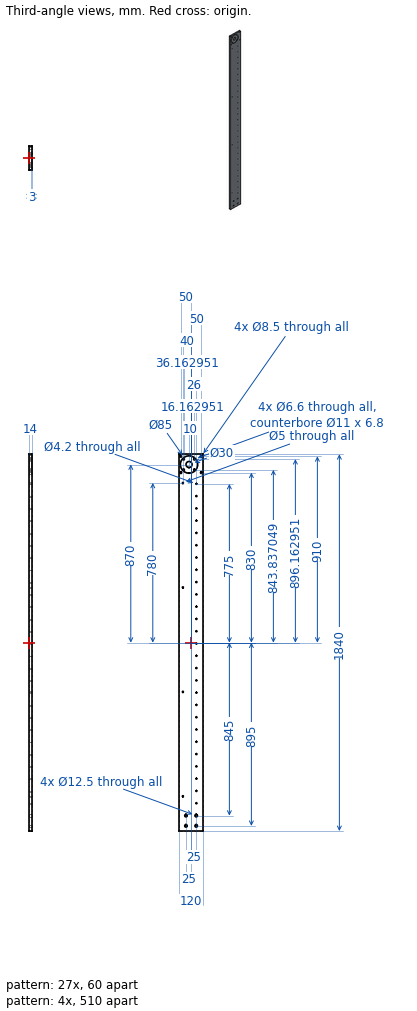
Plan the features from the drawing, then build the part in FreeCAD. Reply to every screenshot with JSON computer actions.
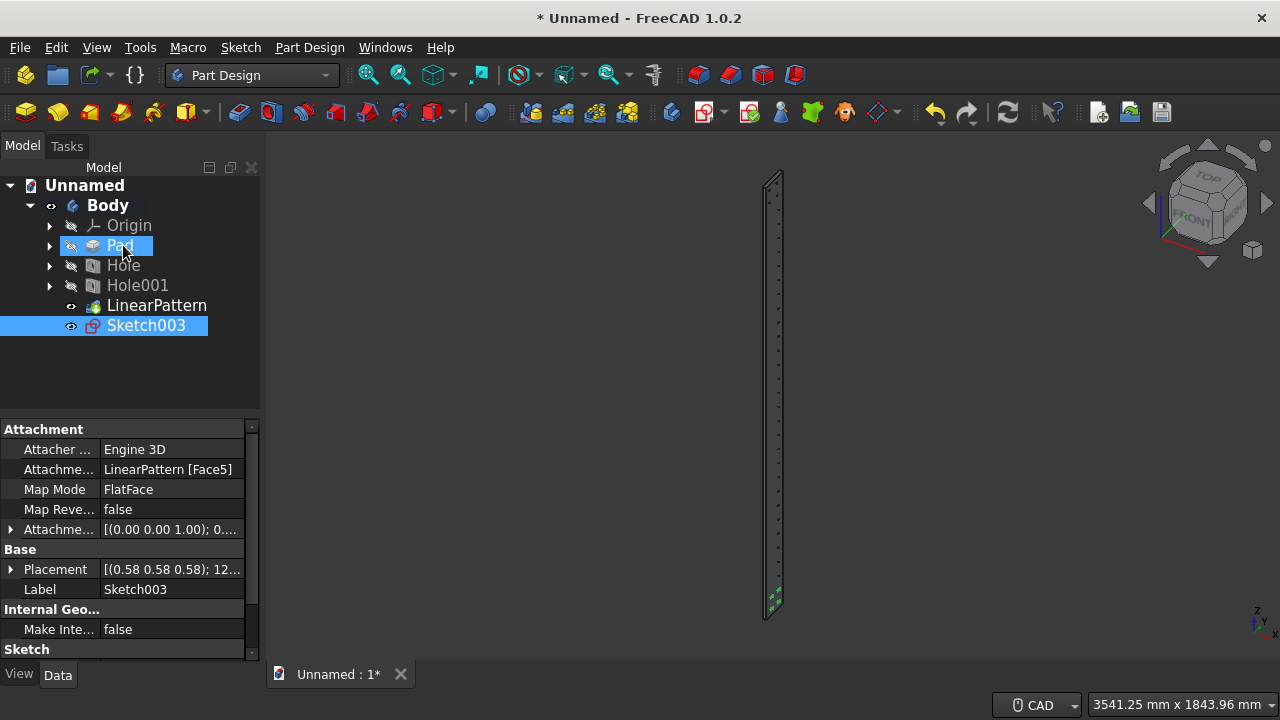
{"action": "left_click", "coordinate": [272, 112]}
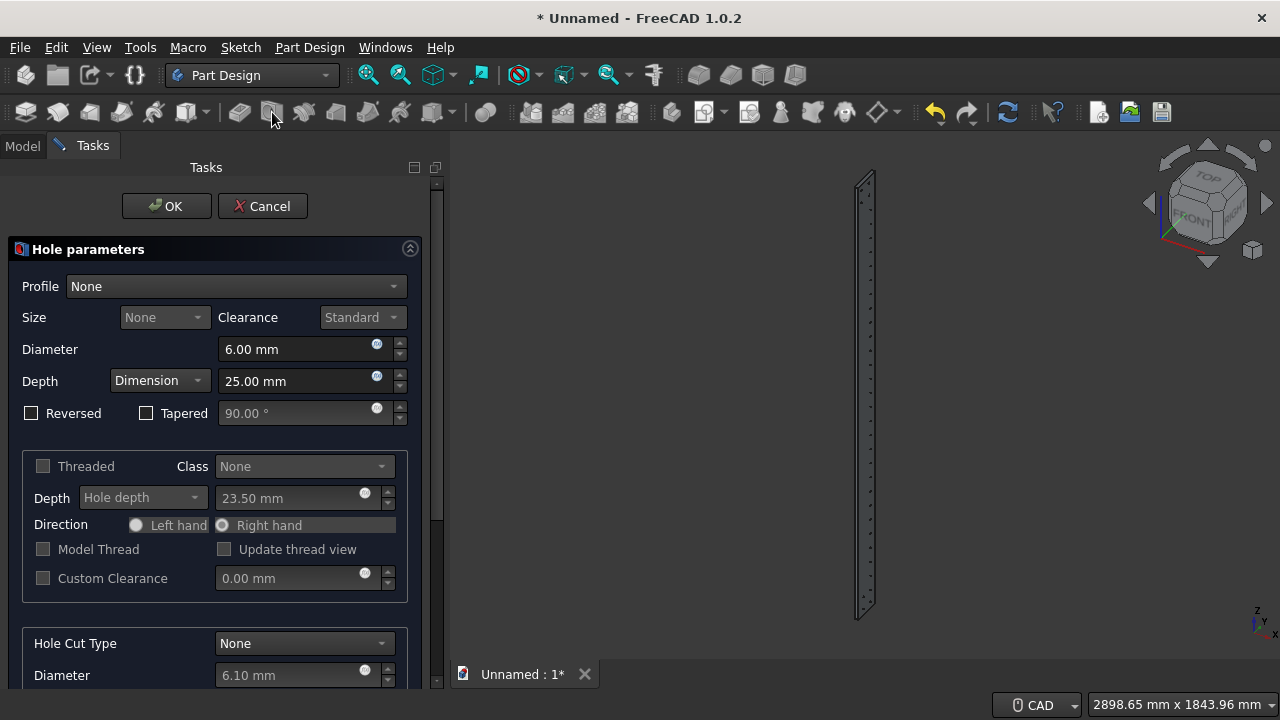
{"action": "triple_click", "coordinate": [305, 349]}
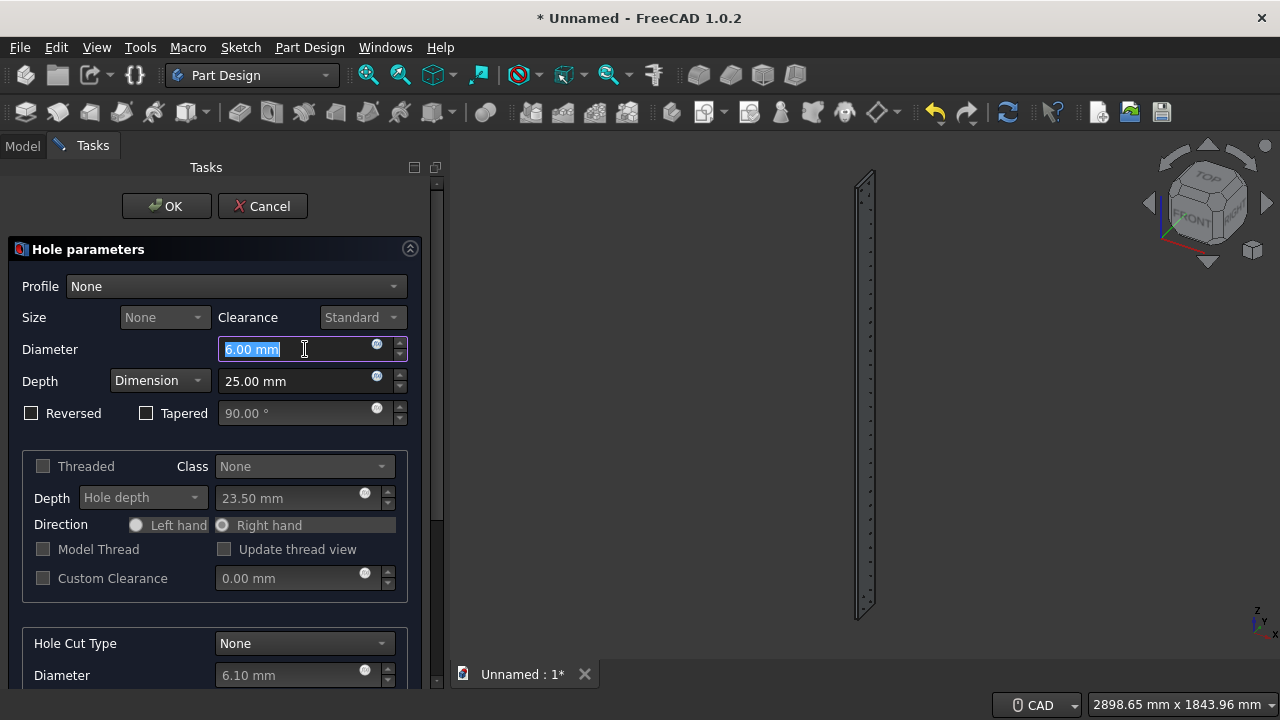
{"action": "type", "text": "12.5"}
{"action": "key", "text": "Tab"}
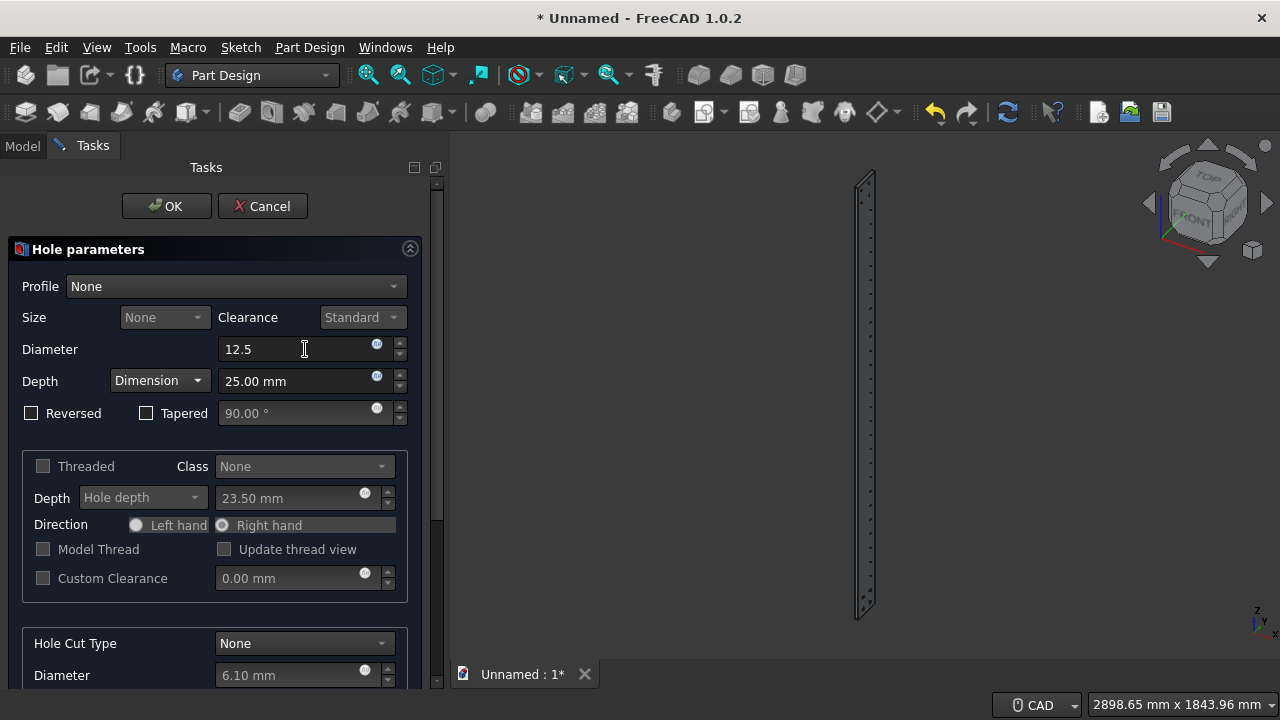
{"action": "left_click", "coordinate": [161, 380]}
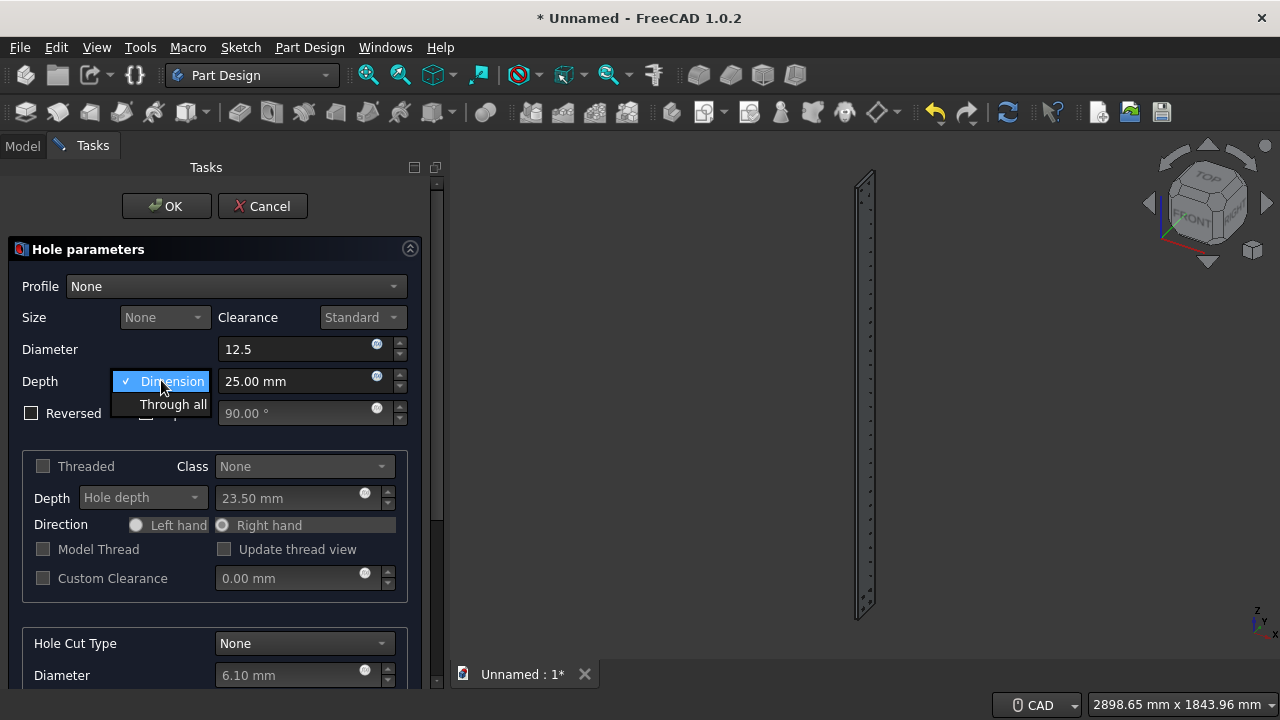
{"action": "left_click", "coordinate": [160, 404]}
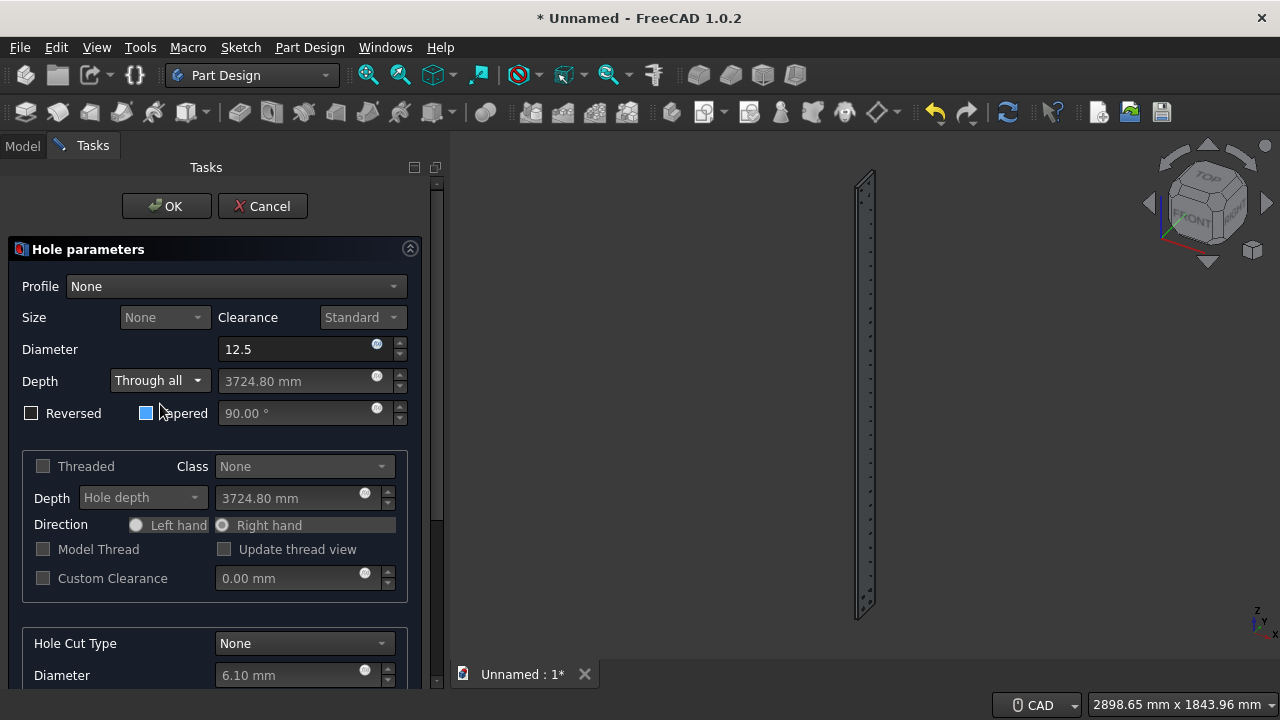
{"action": "left_click", "coordinate": [167, 206]}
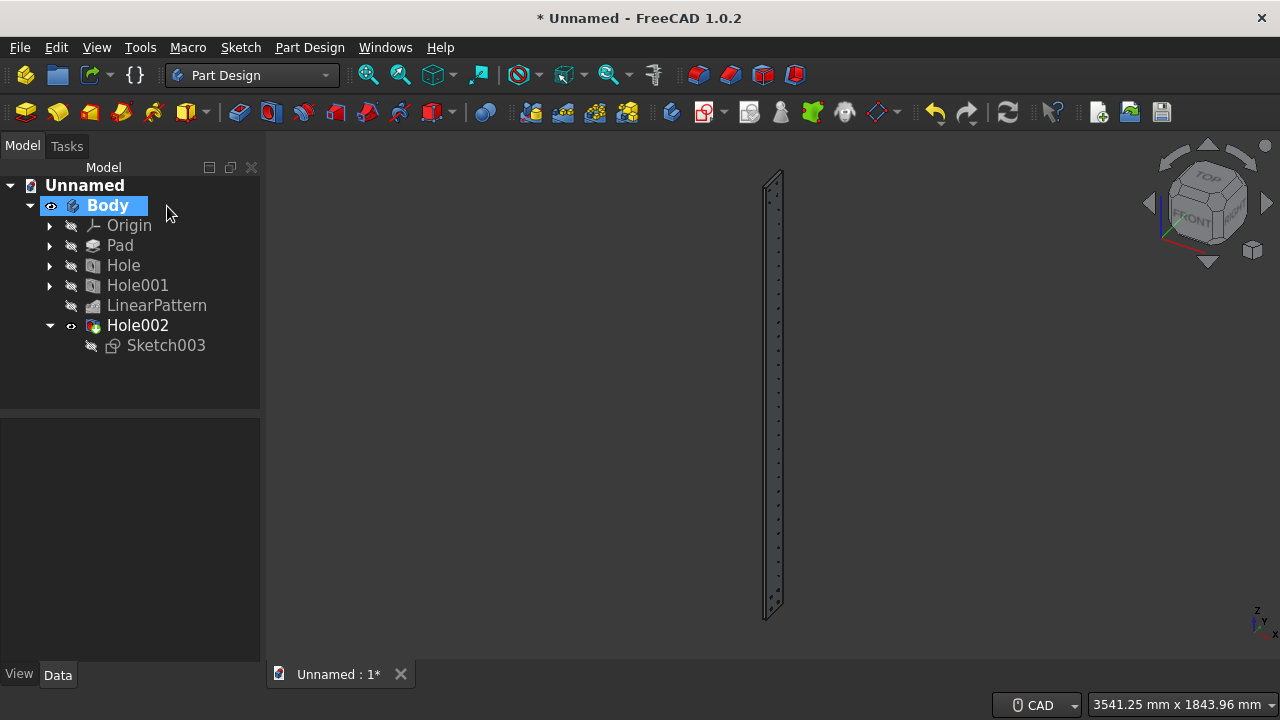
{"action": "left_click", "coordinate": [775, 333]}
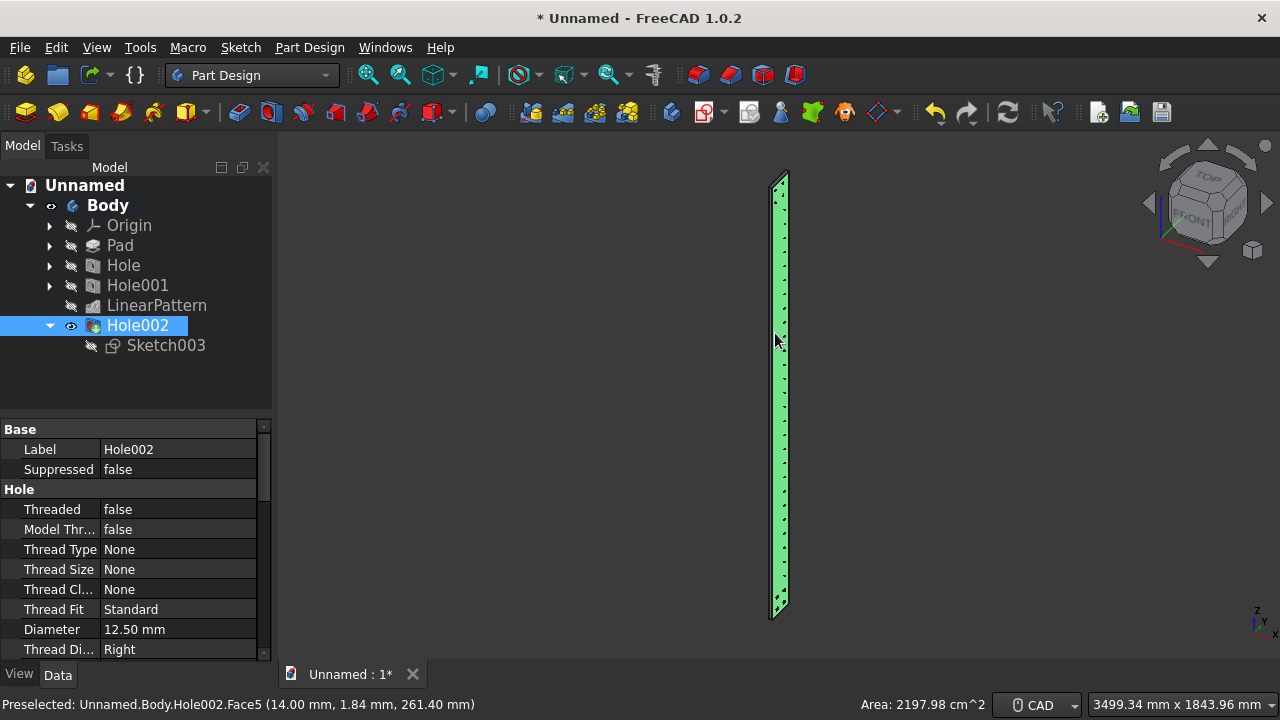
{"action": "left_click", "coordinate": [704, 112]}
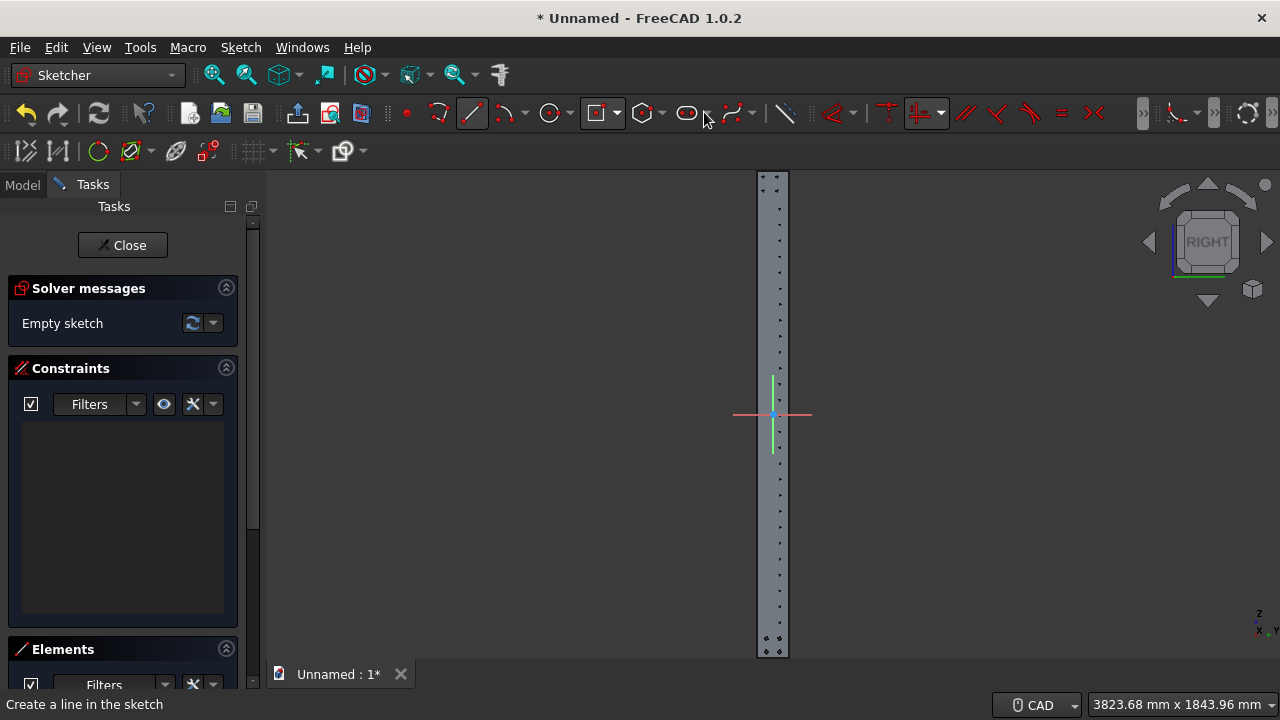
{"action": "scroll", "coordinate": [704, 414], "scroll_direction": "down", "scroll_amount": 5}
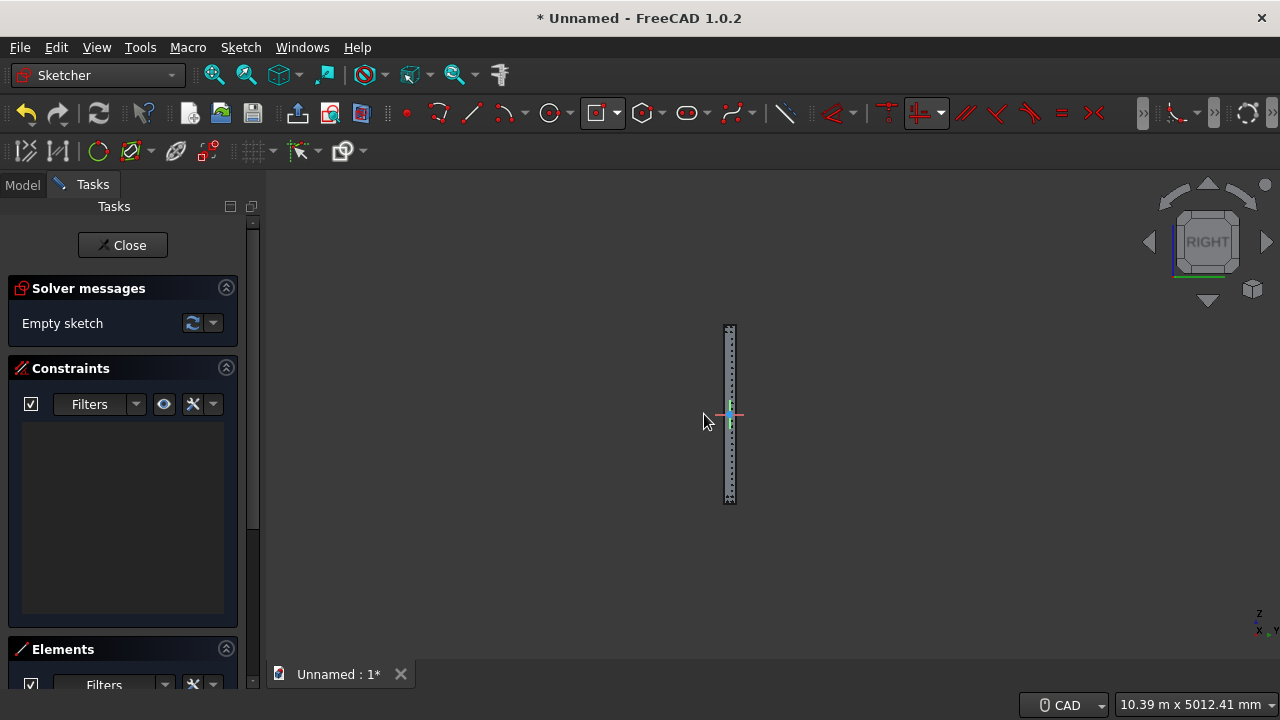
{"action": "scroll", "coordinate": [730, 325], "scroll_direction": "up", "scroll_amount": 15}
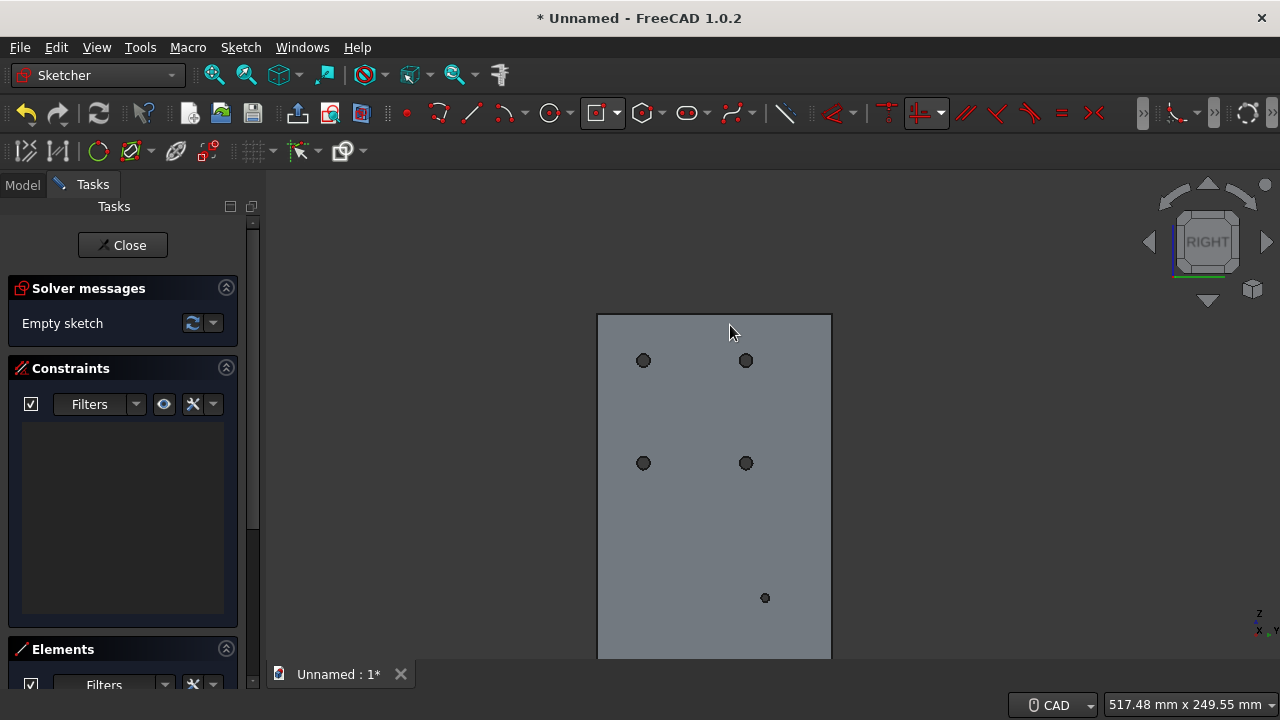
{"action": "scroll", "coordinate": [692, 411], "scroll_direction": "up", "scroll_amount": 8}